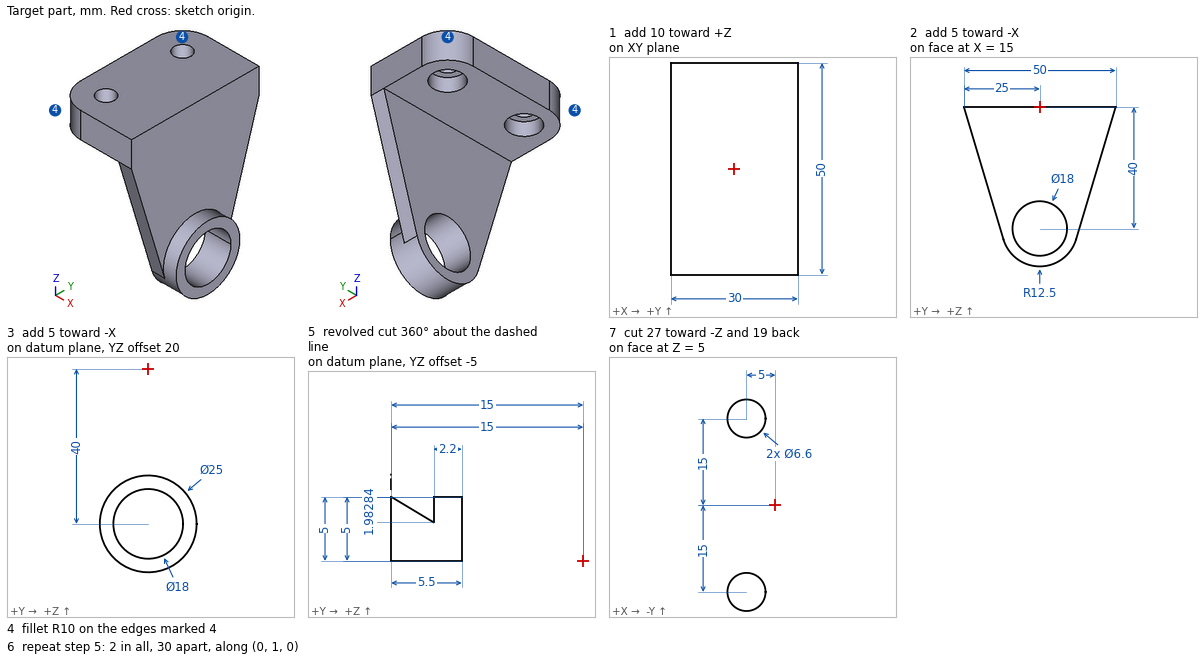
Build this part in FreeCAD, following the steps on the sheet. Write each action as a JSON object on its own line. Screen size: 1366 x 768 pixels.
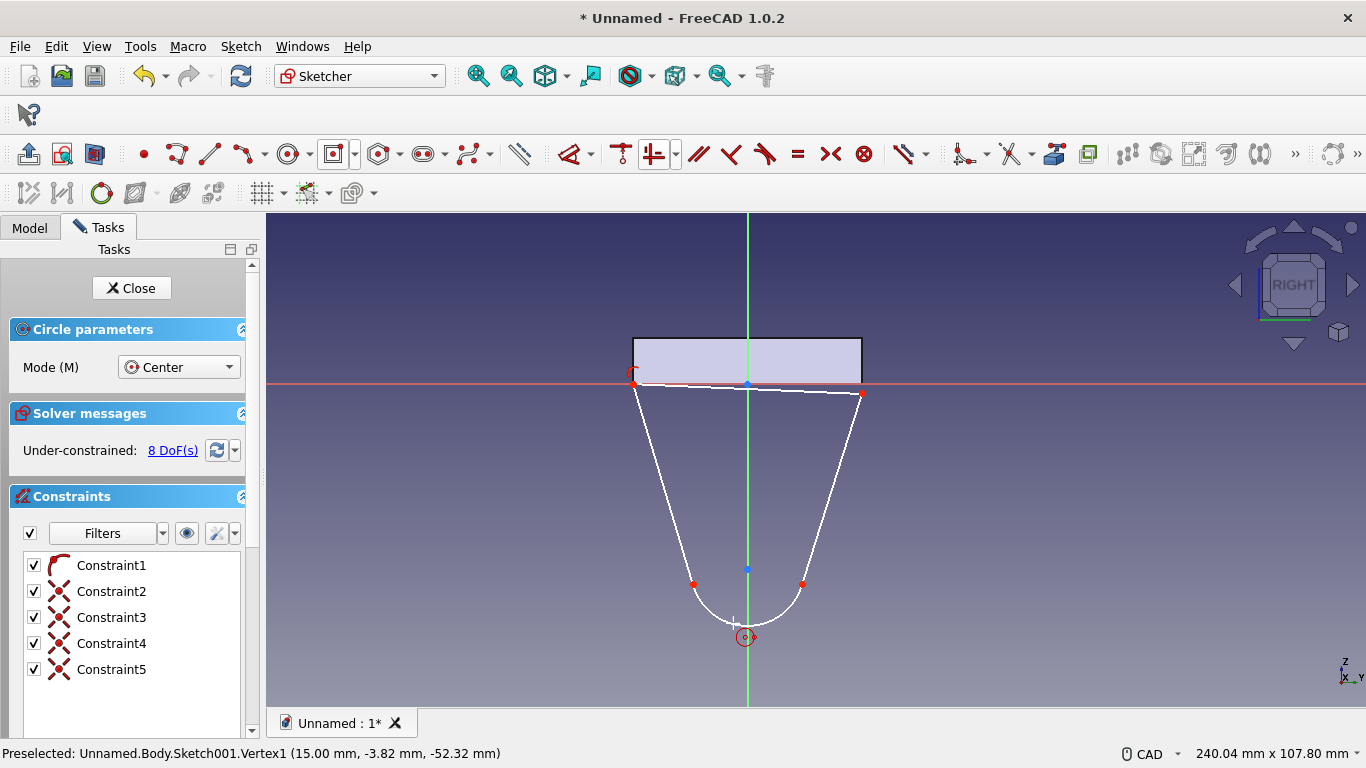
{"action": "left_click", "coordinate": [748, 567]}
{"action": "mouse_move", "coordinate": [777, 538]}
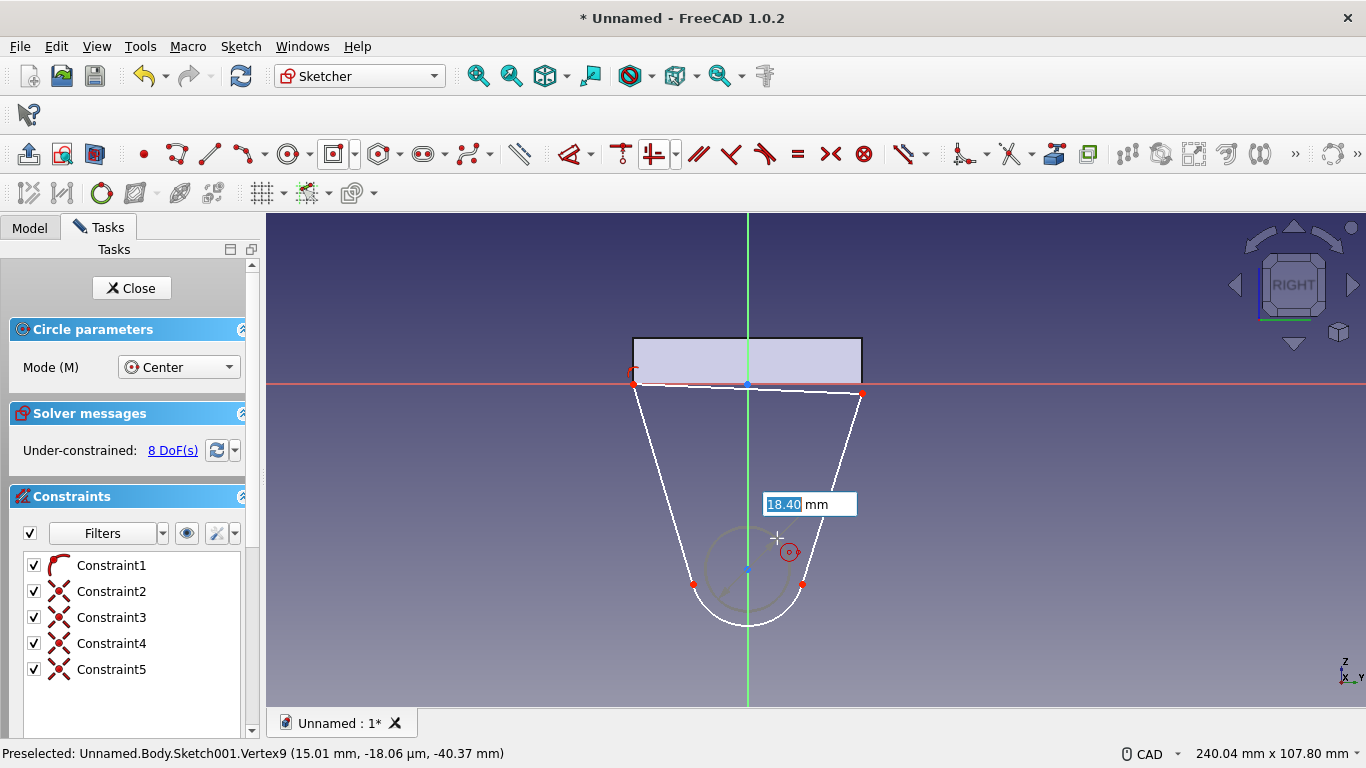
{"action": "type", "text": "18"}
{"action": "key", "text": "Return"}
{"action": "key", "text": "Escape"}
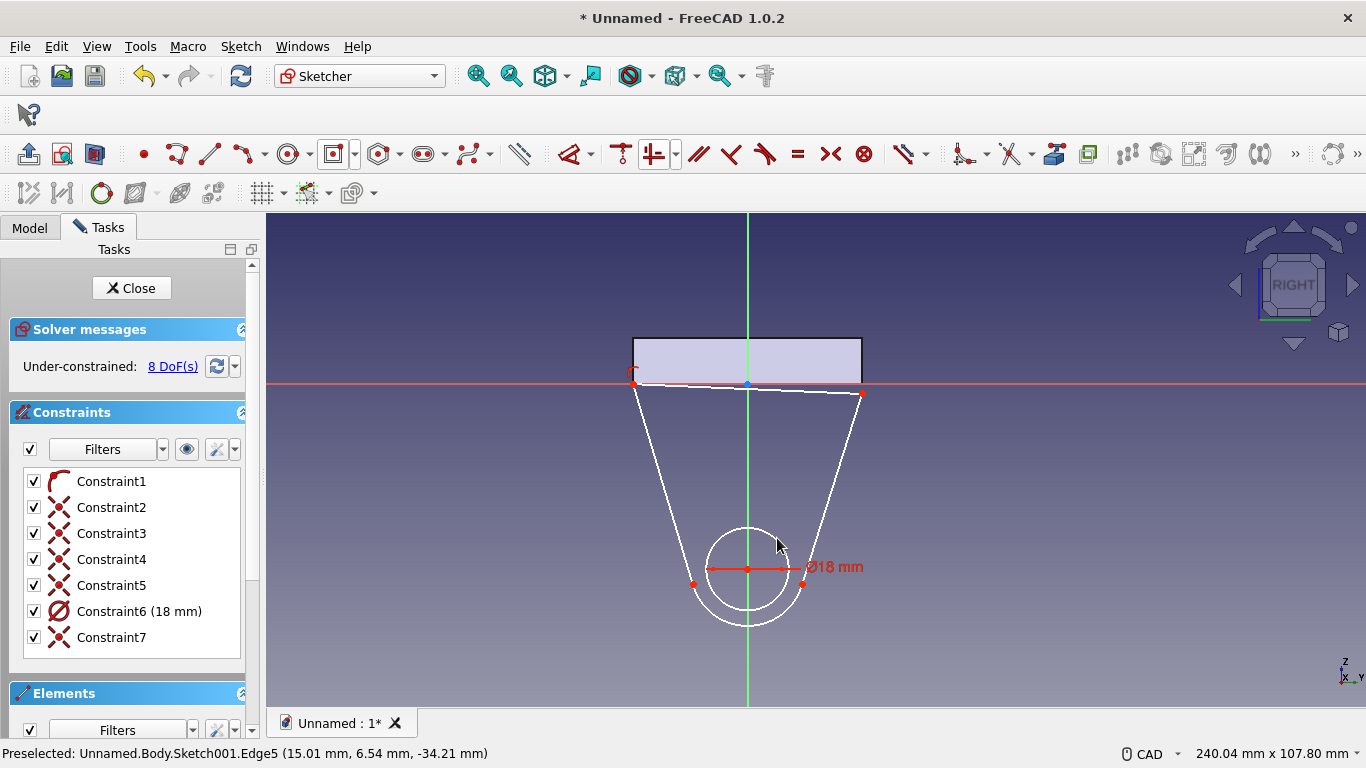
{"action": "left_click", "coordinate": [675, 525]}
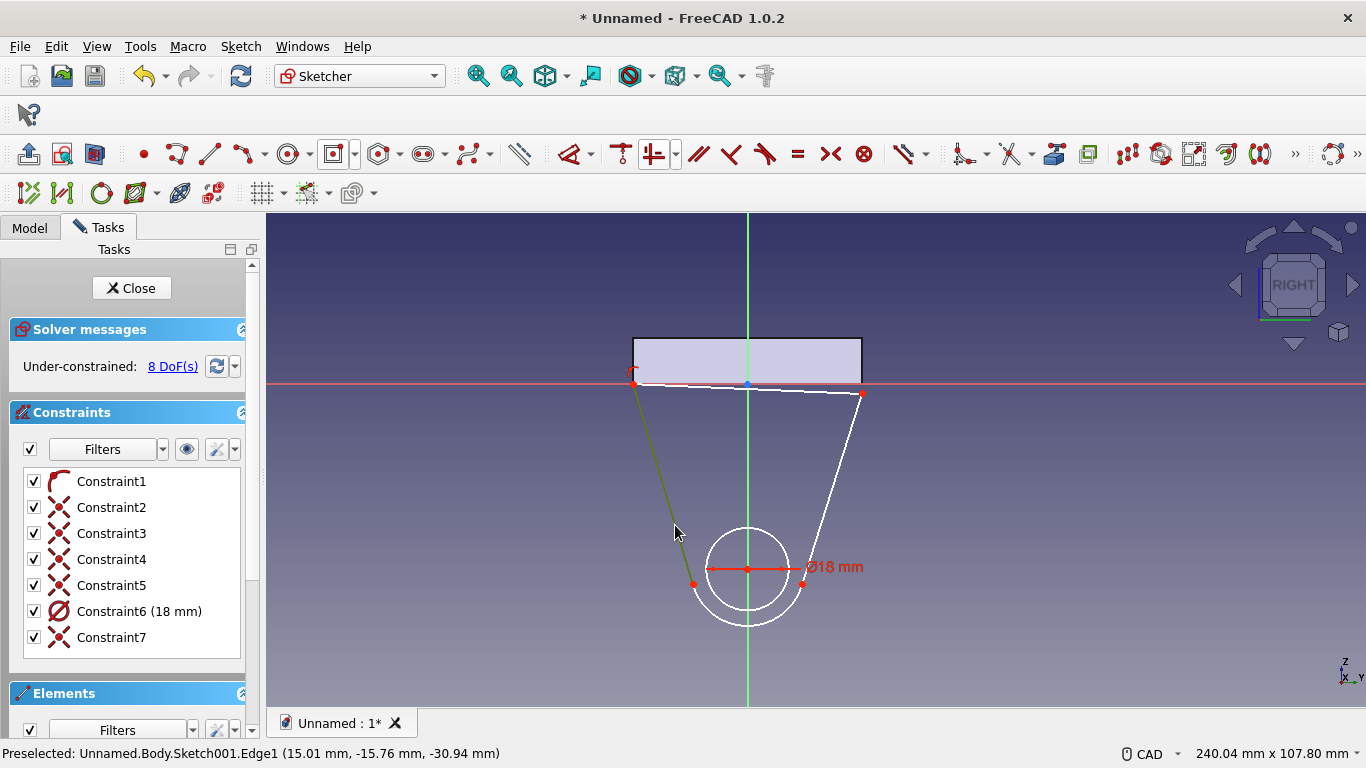
{"action": "left_click", "coordinate": [720, 619]}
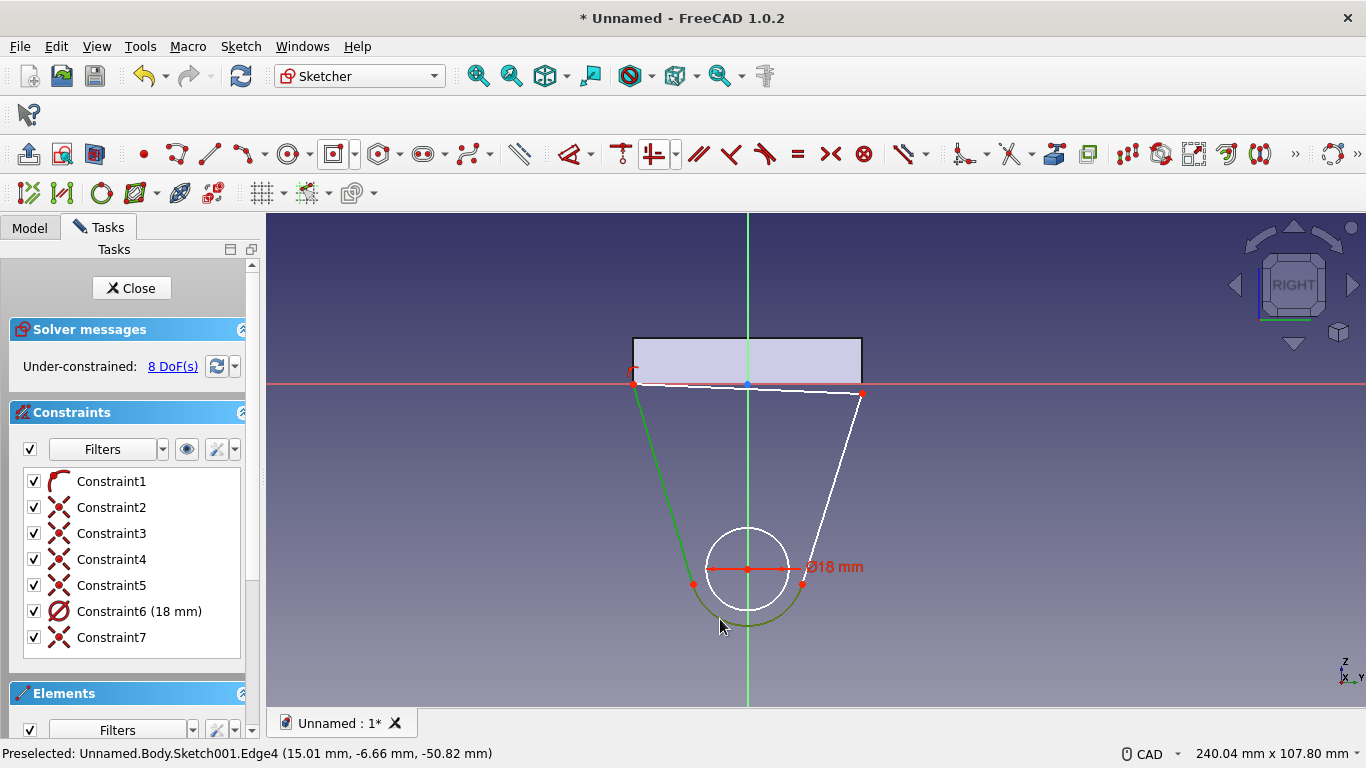
{"action": "left_click", "coordinate": [765, 154]}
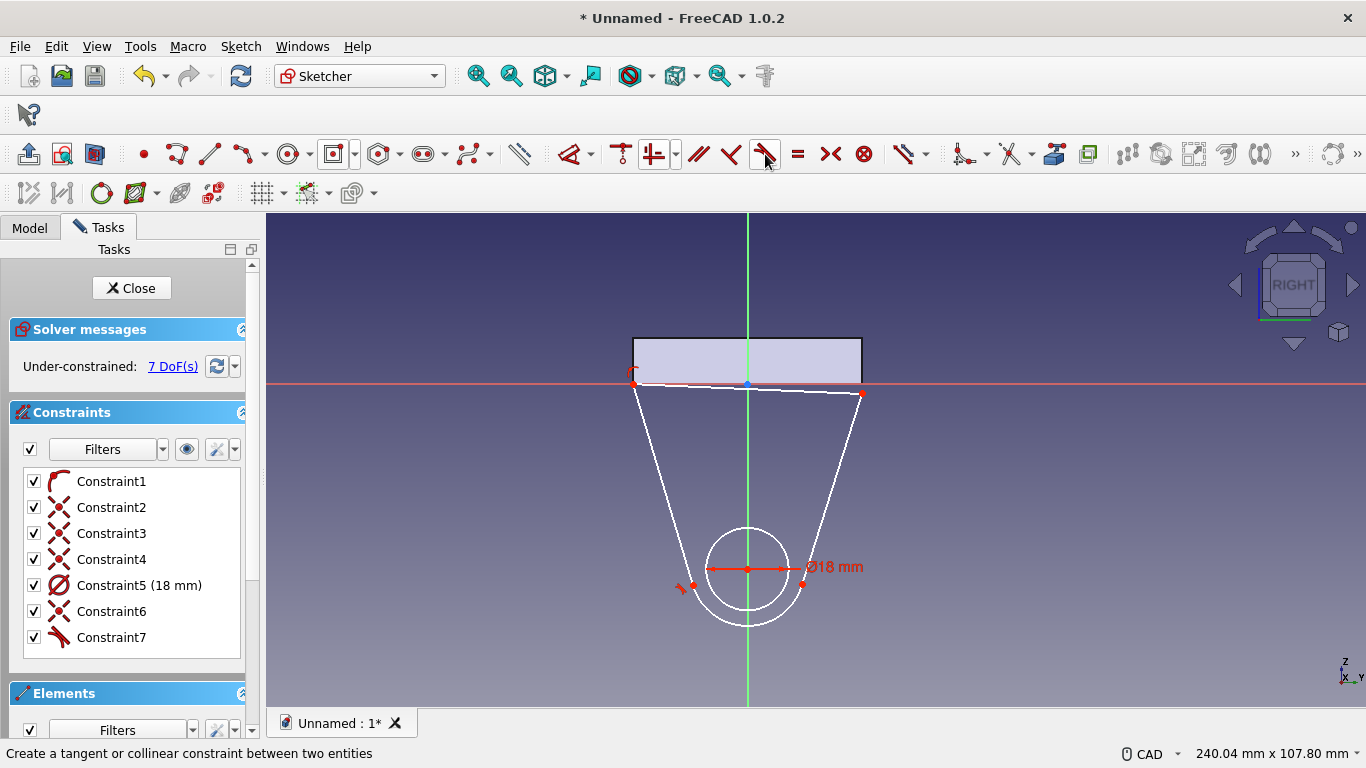
{"action": "left_click", "coordinate": [844, 451]}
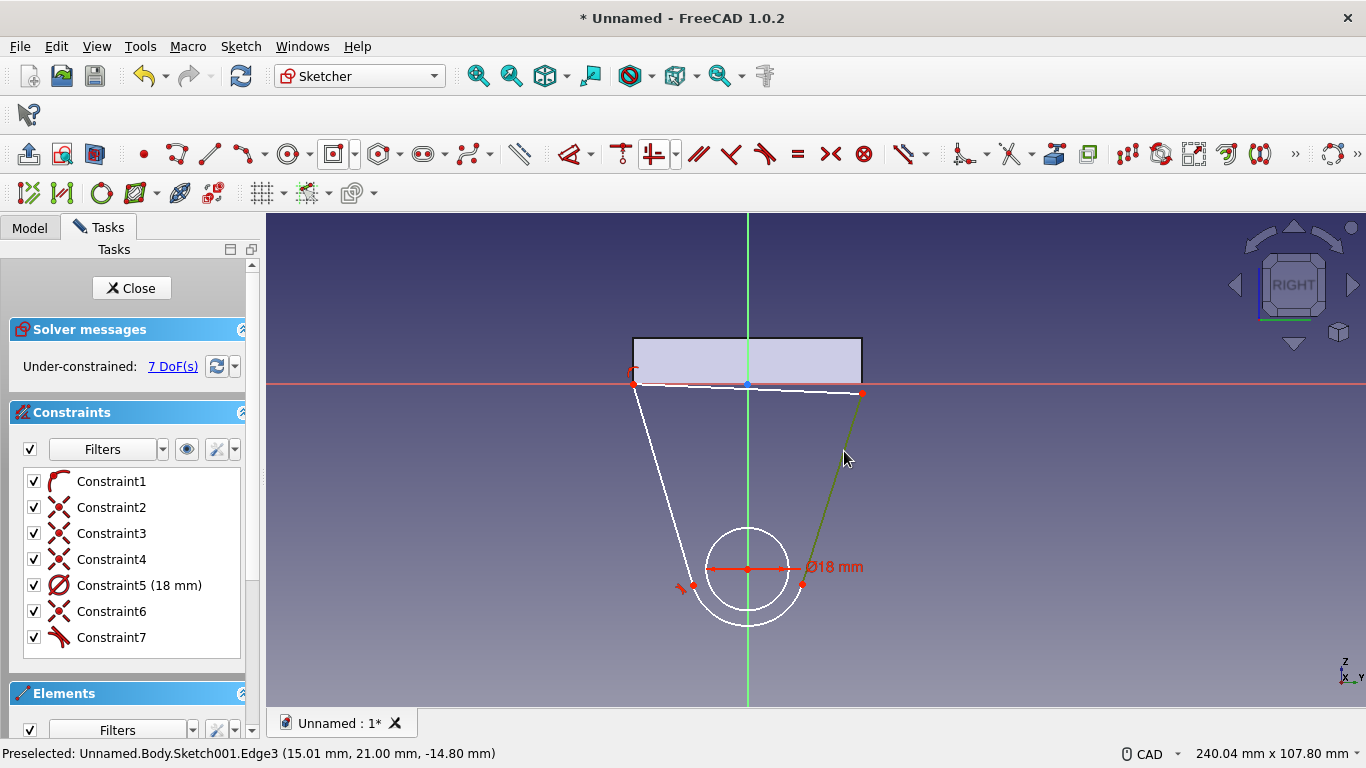
{"action": "left_click", "coordinate": [720, 619]}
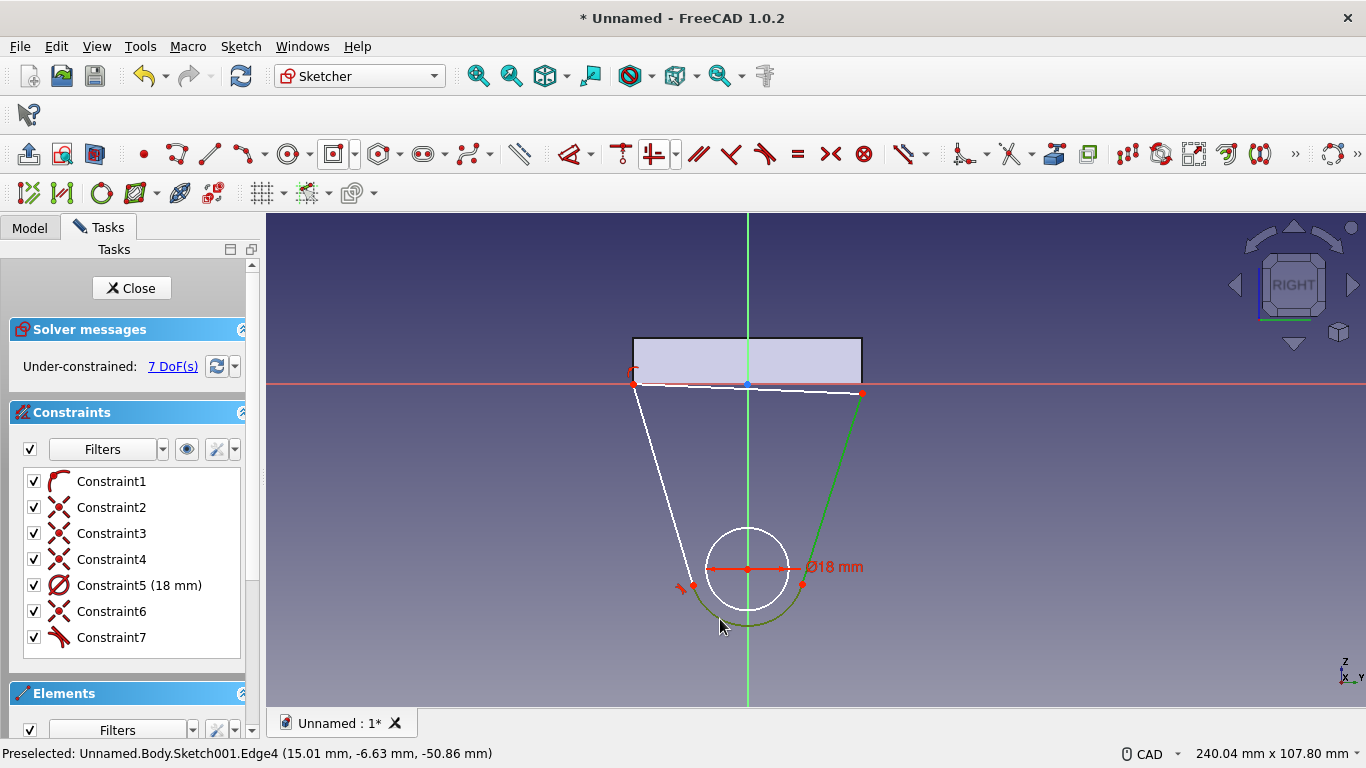
{"action": "left_click", "coordinate": [765, 154]}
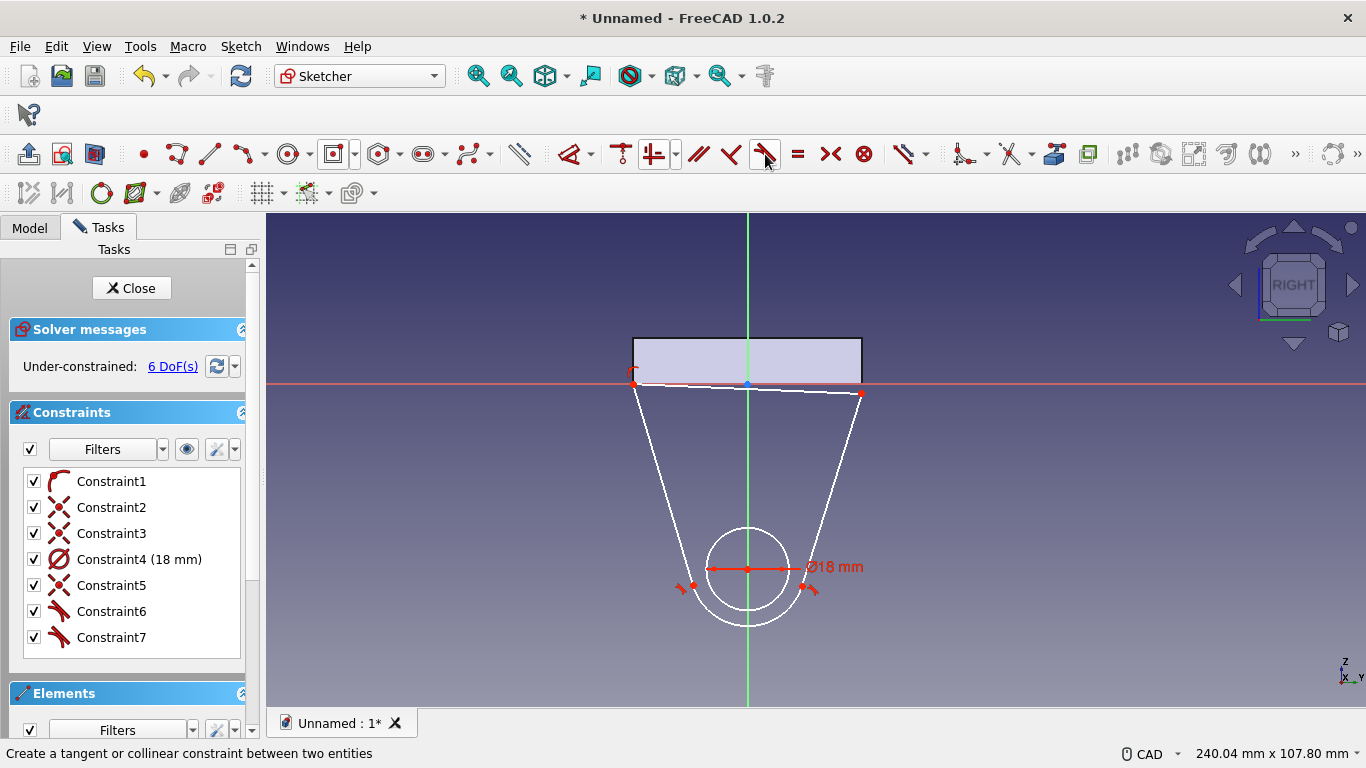
{"action": "left_click", "coordinate": [702, 387]}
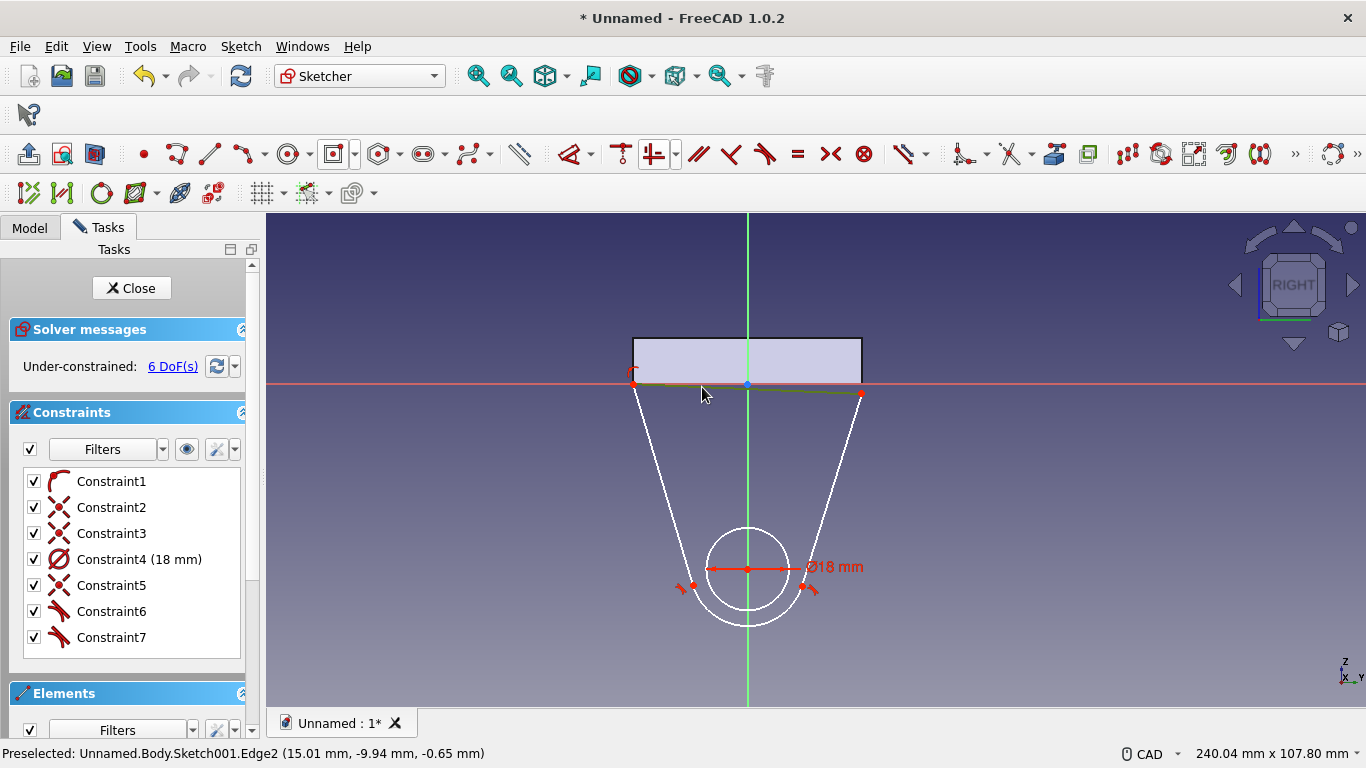
{"action": "key", "text": "h"}